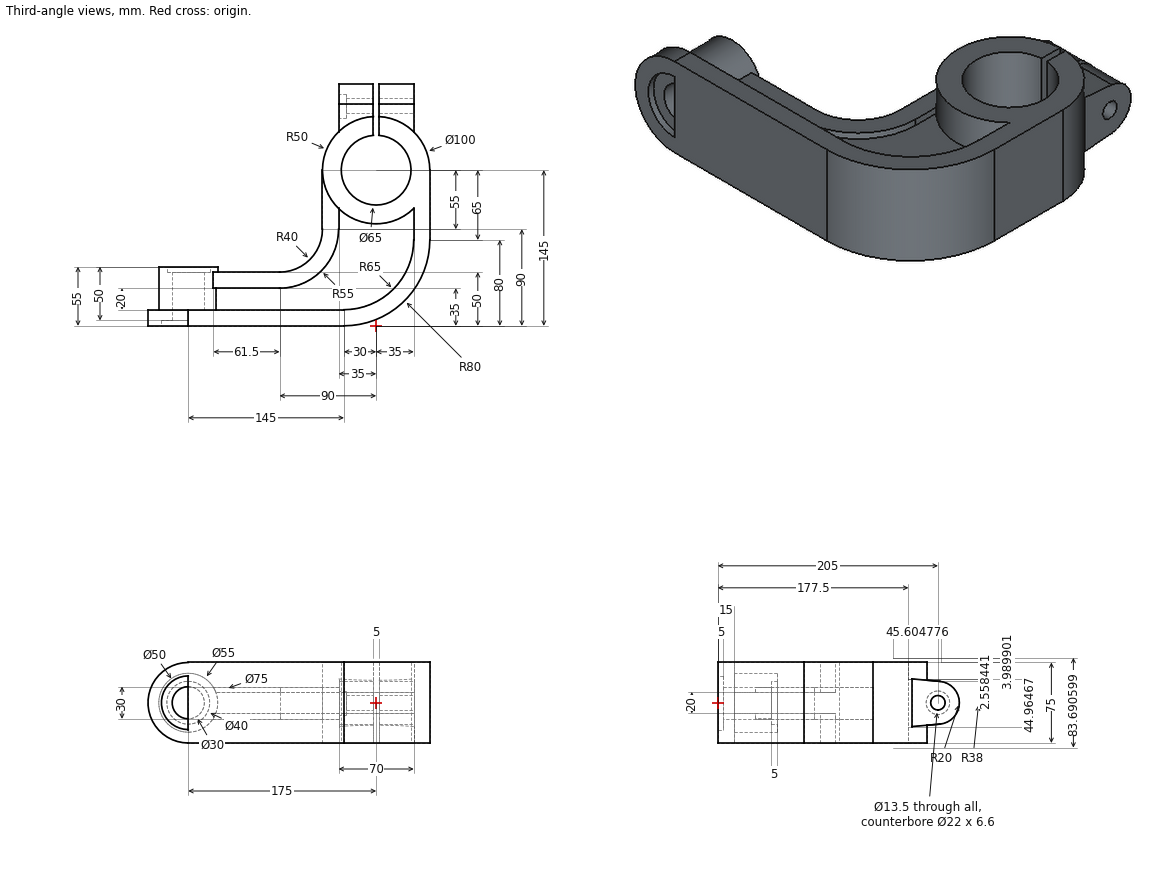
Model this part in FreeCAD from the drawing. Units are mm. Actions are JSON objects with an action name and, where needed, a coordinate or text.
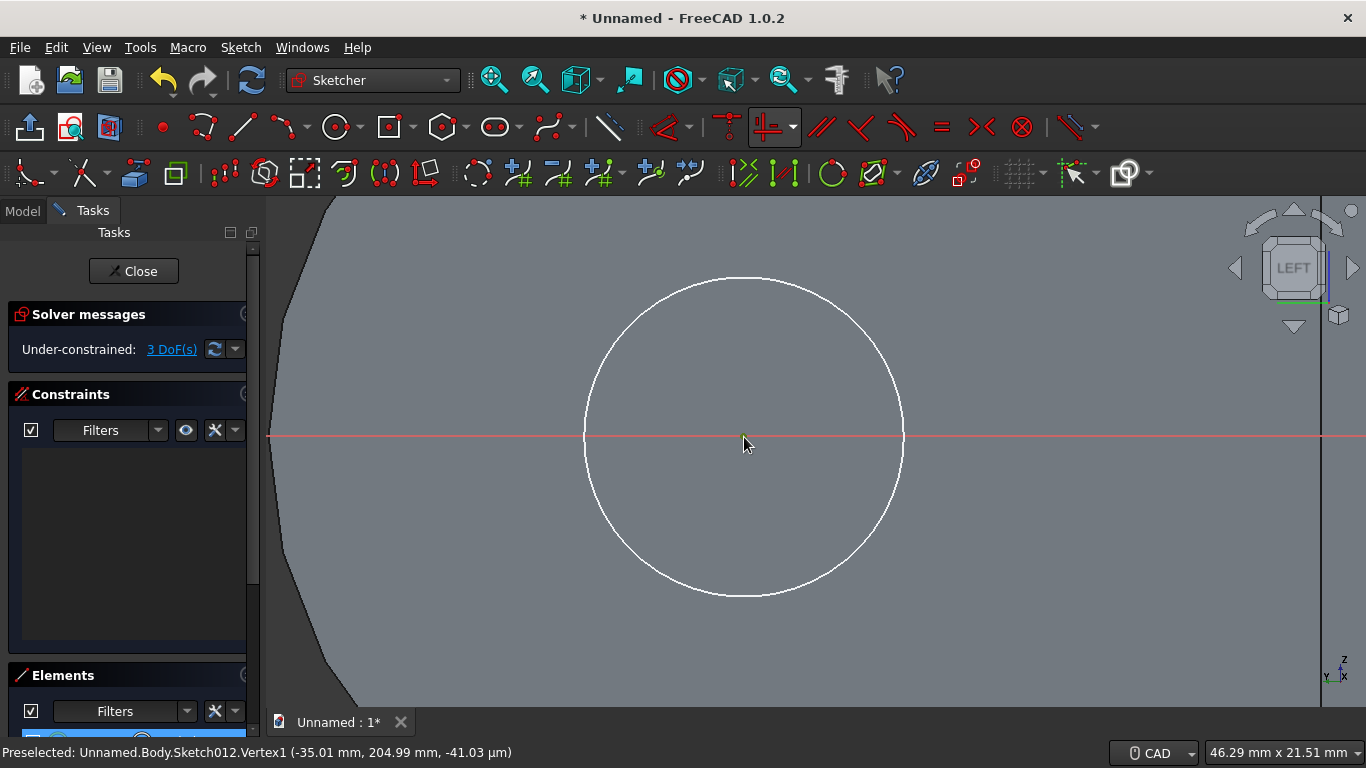
{"action": "left_click", "coordinate": [359, 436]}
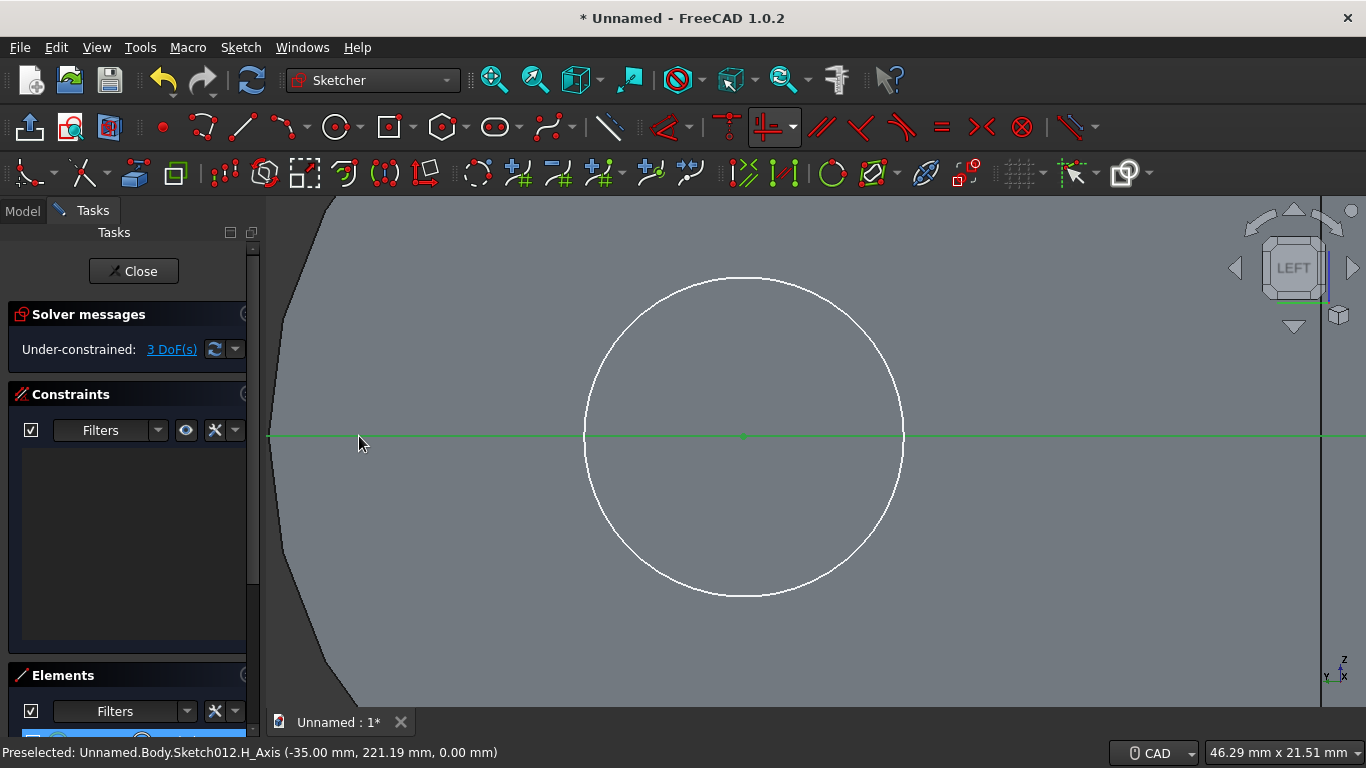
{"action": "key", "text": "c"}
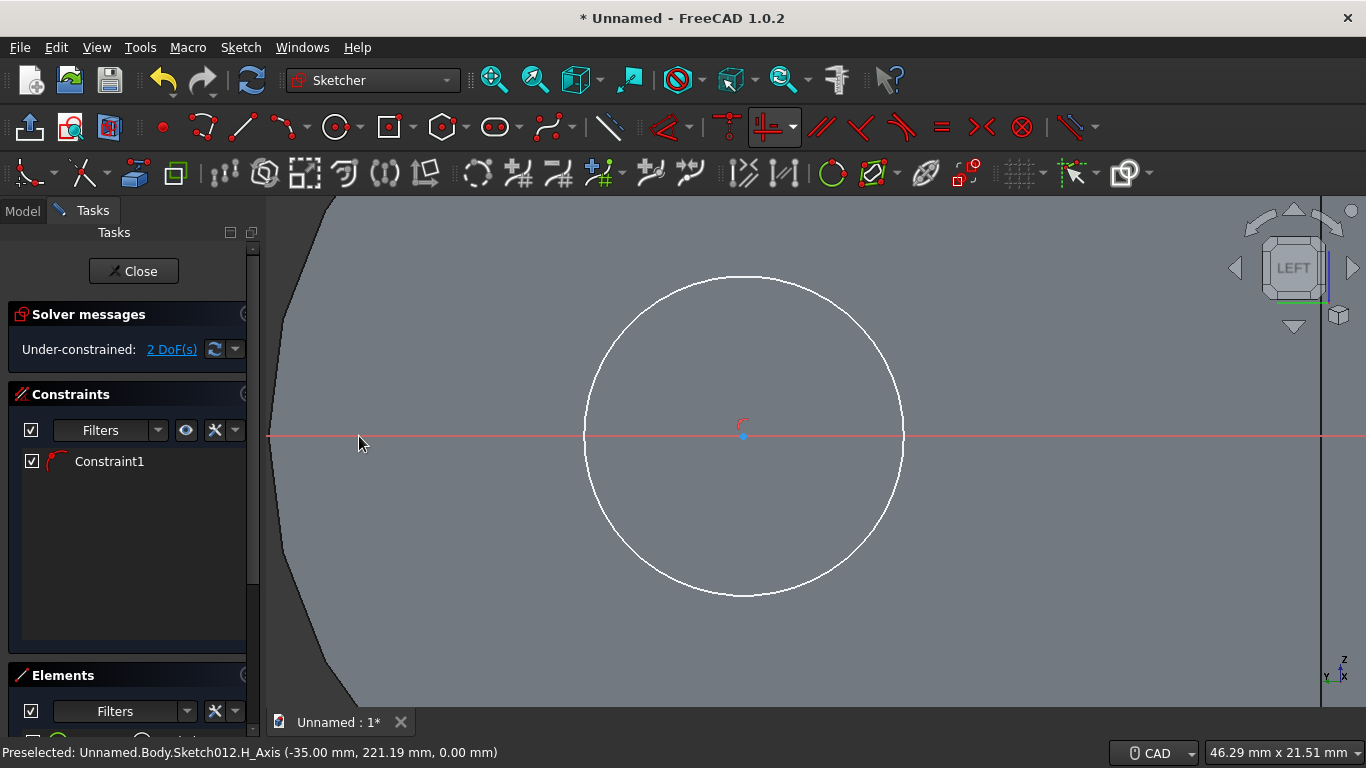
{"action": "key", "text": "d"}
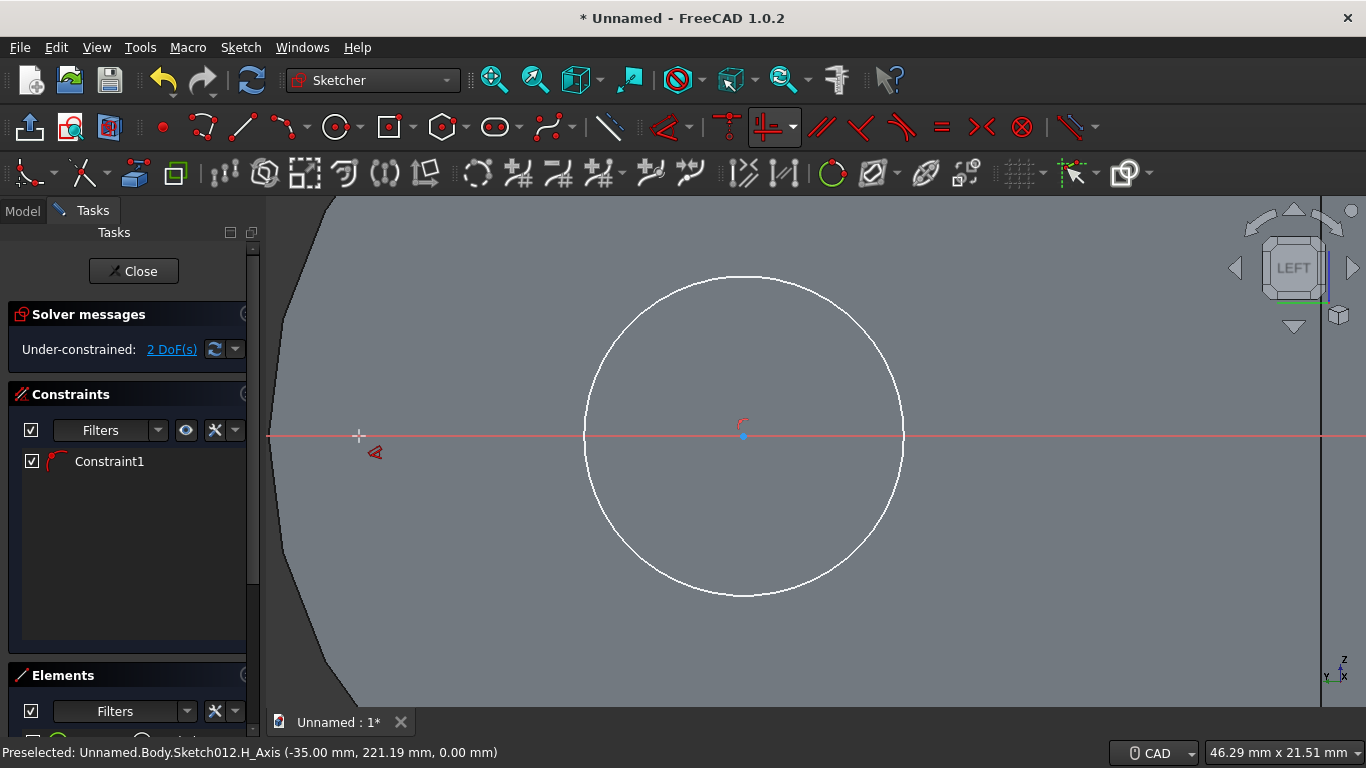
{"action": "left_click", "coordinate": [857, 323]}
{"action": "left_click", "coordinate": [880, 300]}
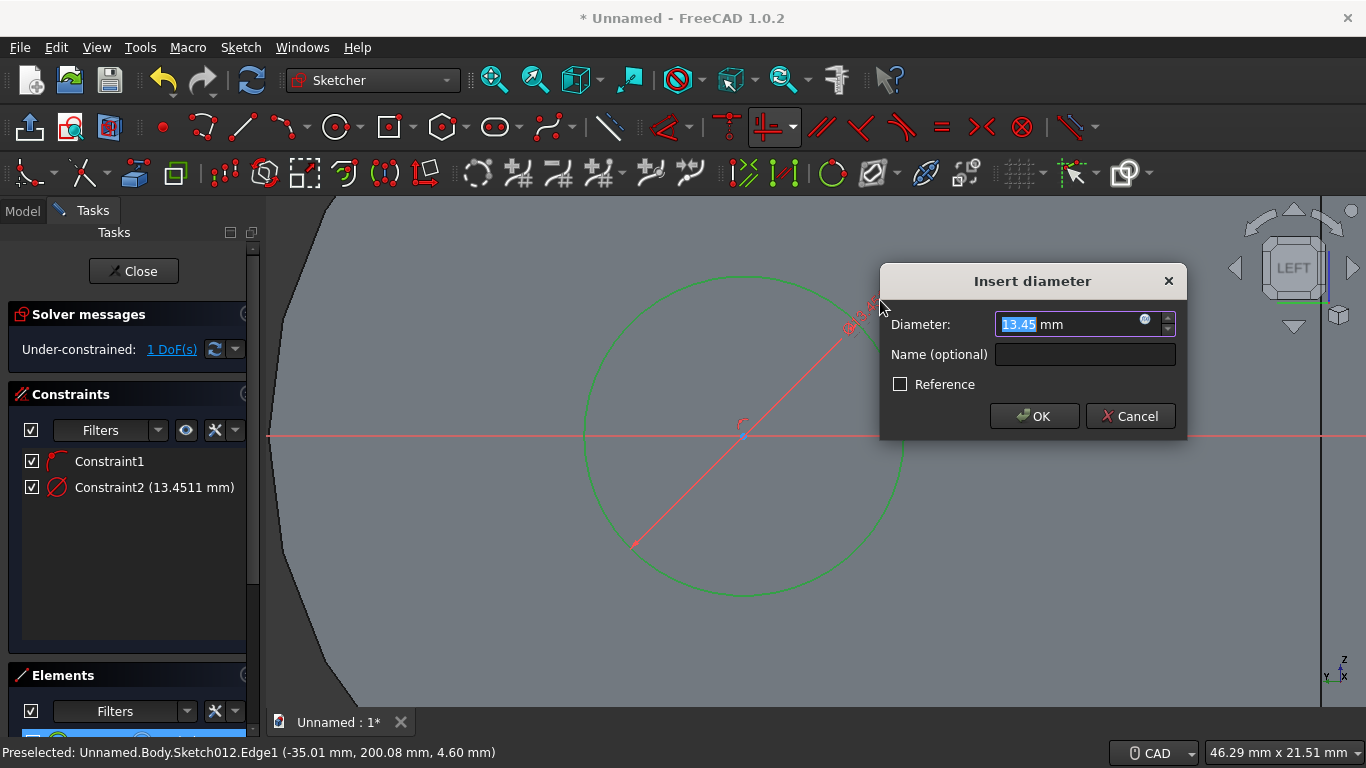
{"action": "type", "text": "13.5"}
{"action": "key", "text": "Return"}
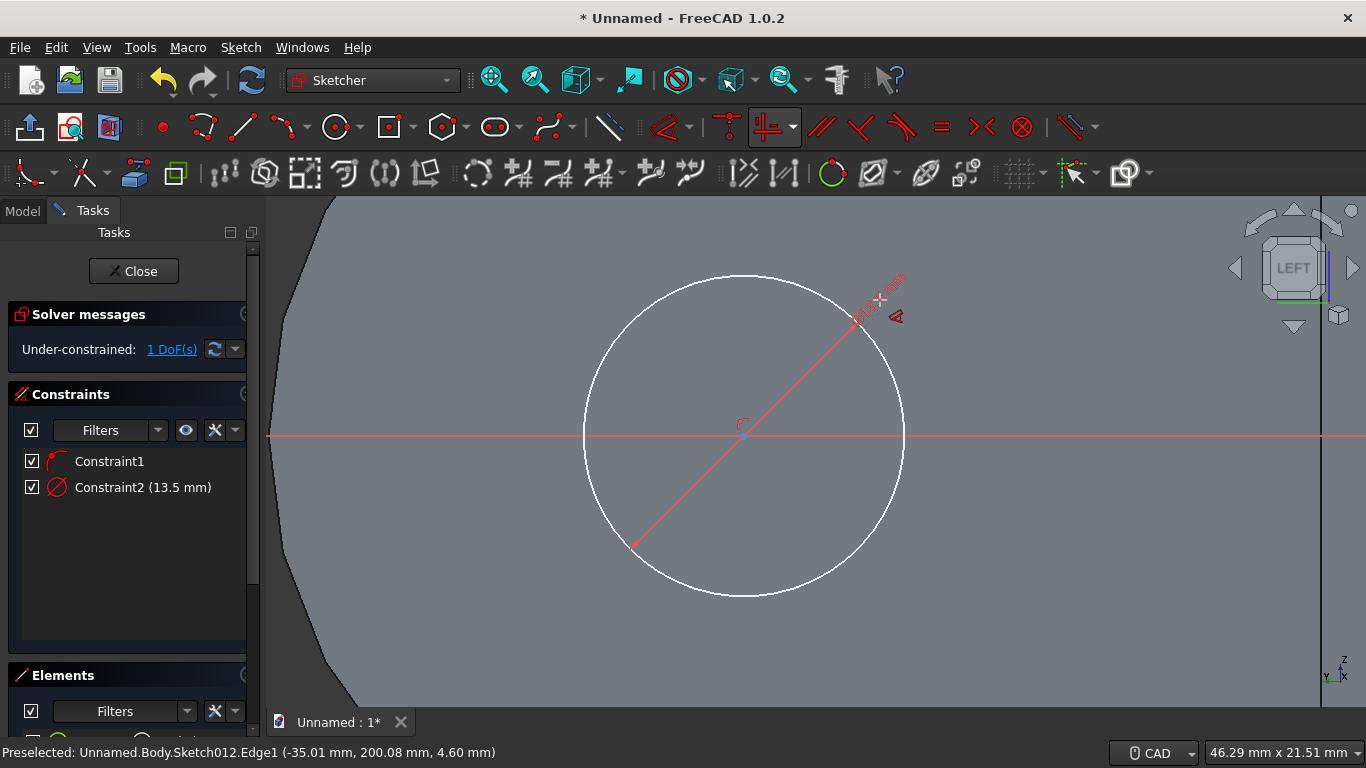
{"action": "left_click", "coordinate": [744, 436]}
{"action": "left_click", "coordinate": [972, 470]}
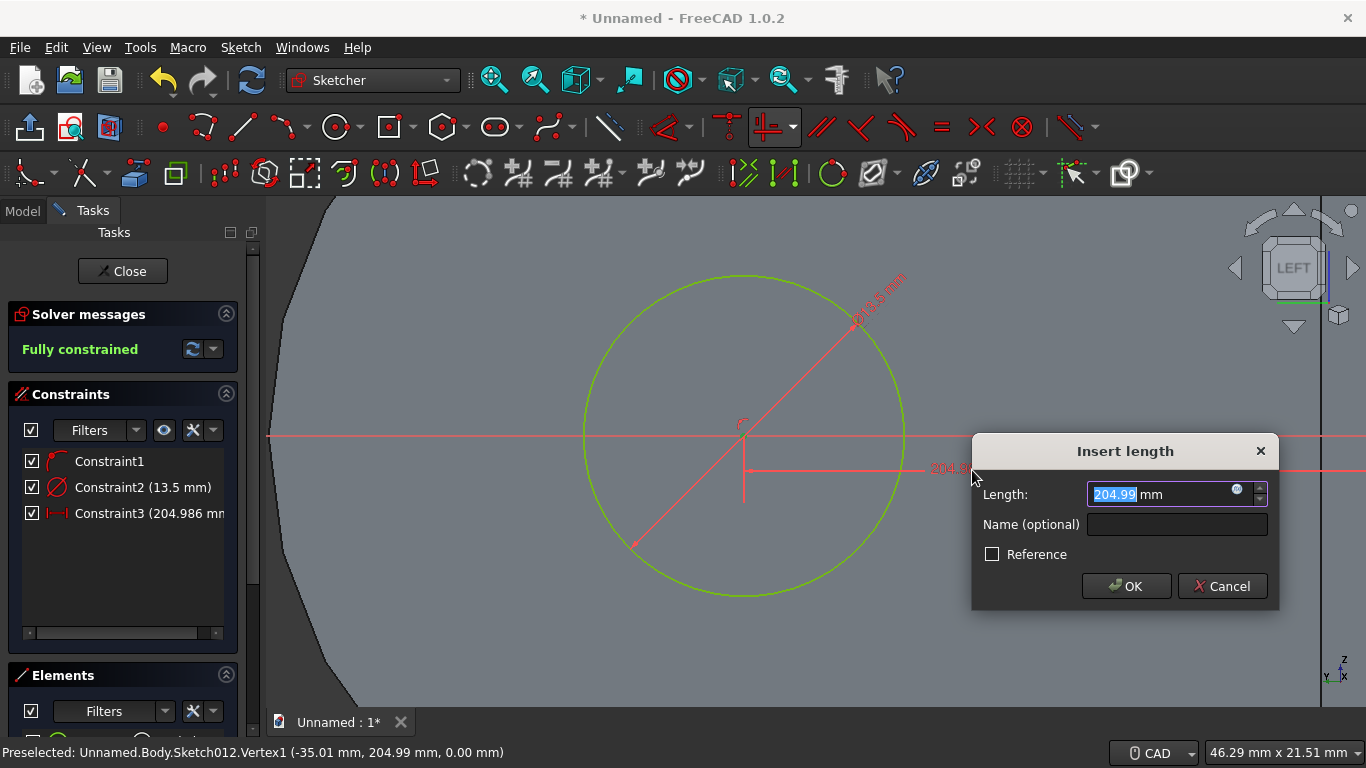
{"action": "type", "text": "205"}
{"action": "key", "text": "Return"}
{"action": "key", "text": "Escape"}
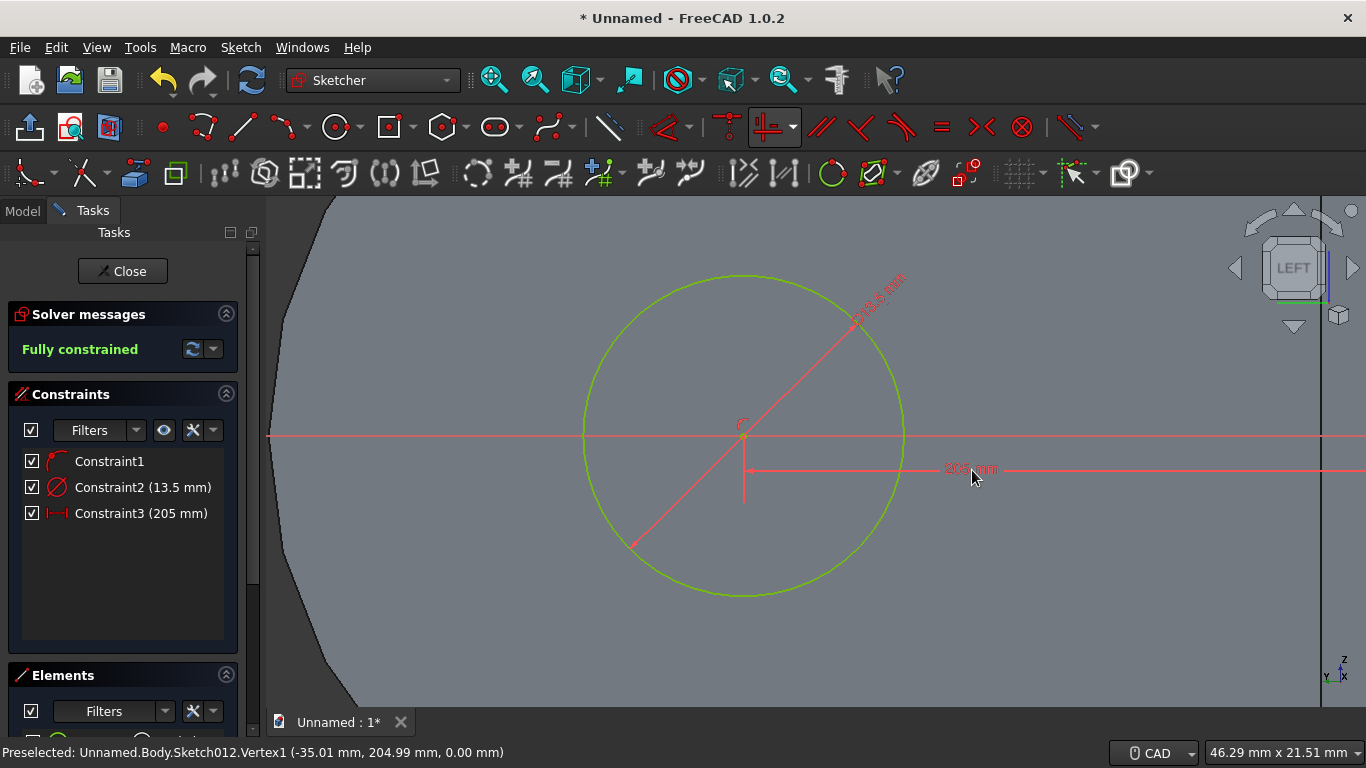
{"action": "left_click", "coordinate": [123, 271]}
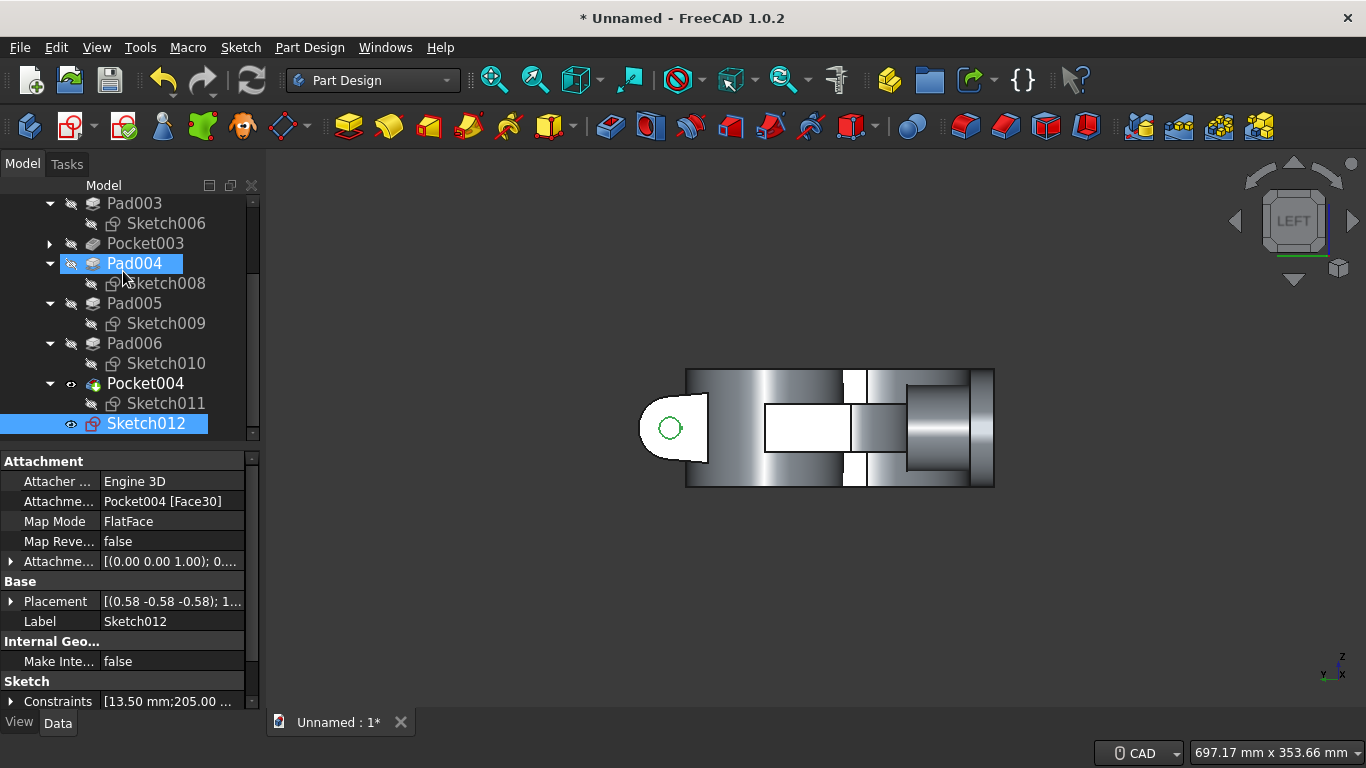
{"action": "left_click", "coordinate": [652, 126]}